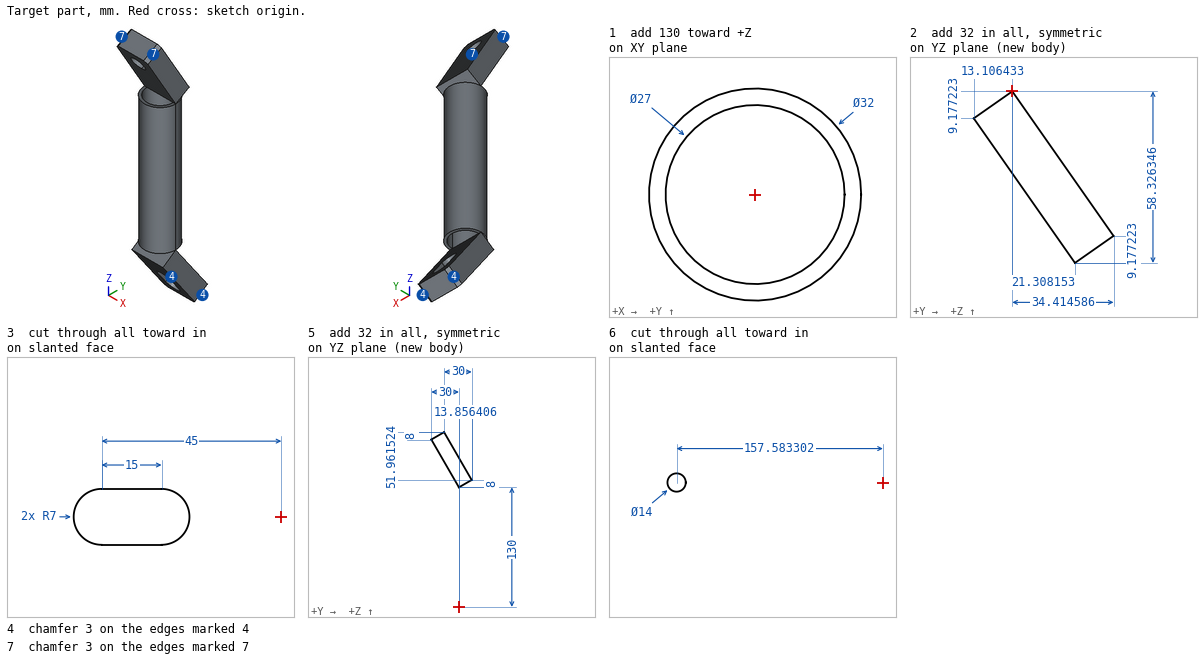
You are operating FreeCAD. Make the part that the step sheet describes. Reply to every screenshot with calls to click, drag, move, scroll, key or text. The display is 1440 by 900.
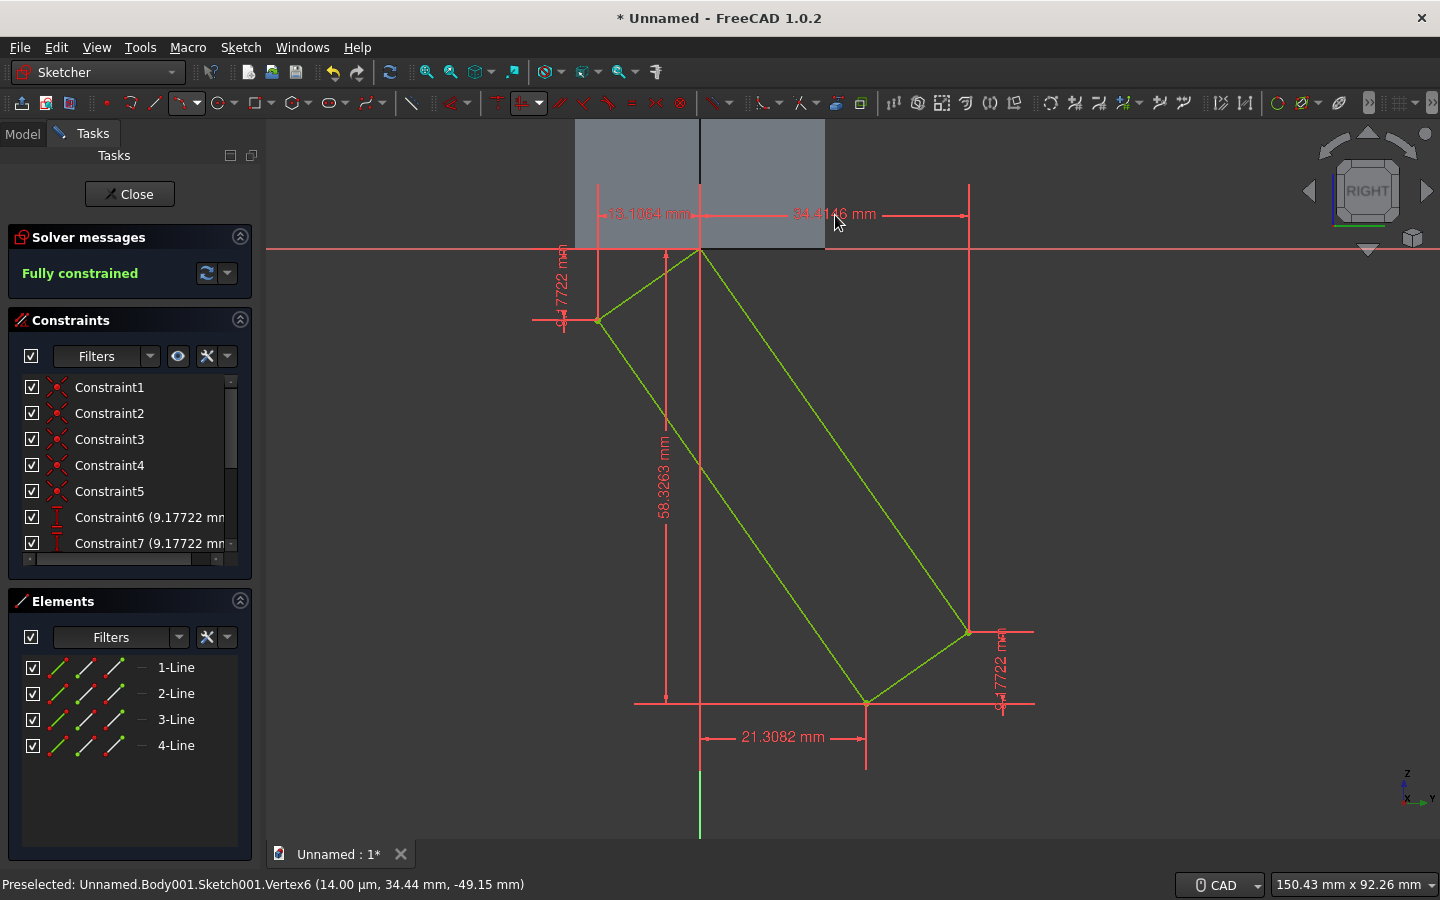
click(130, 194)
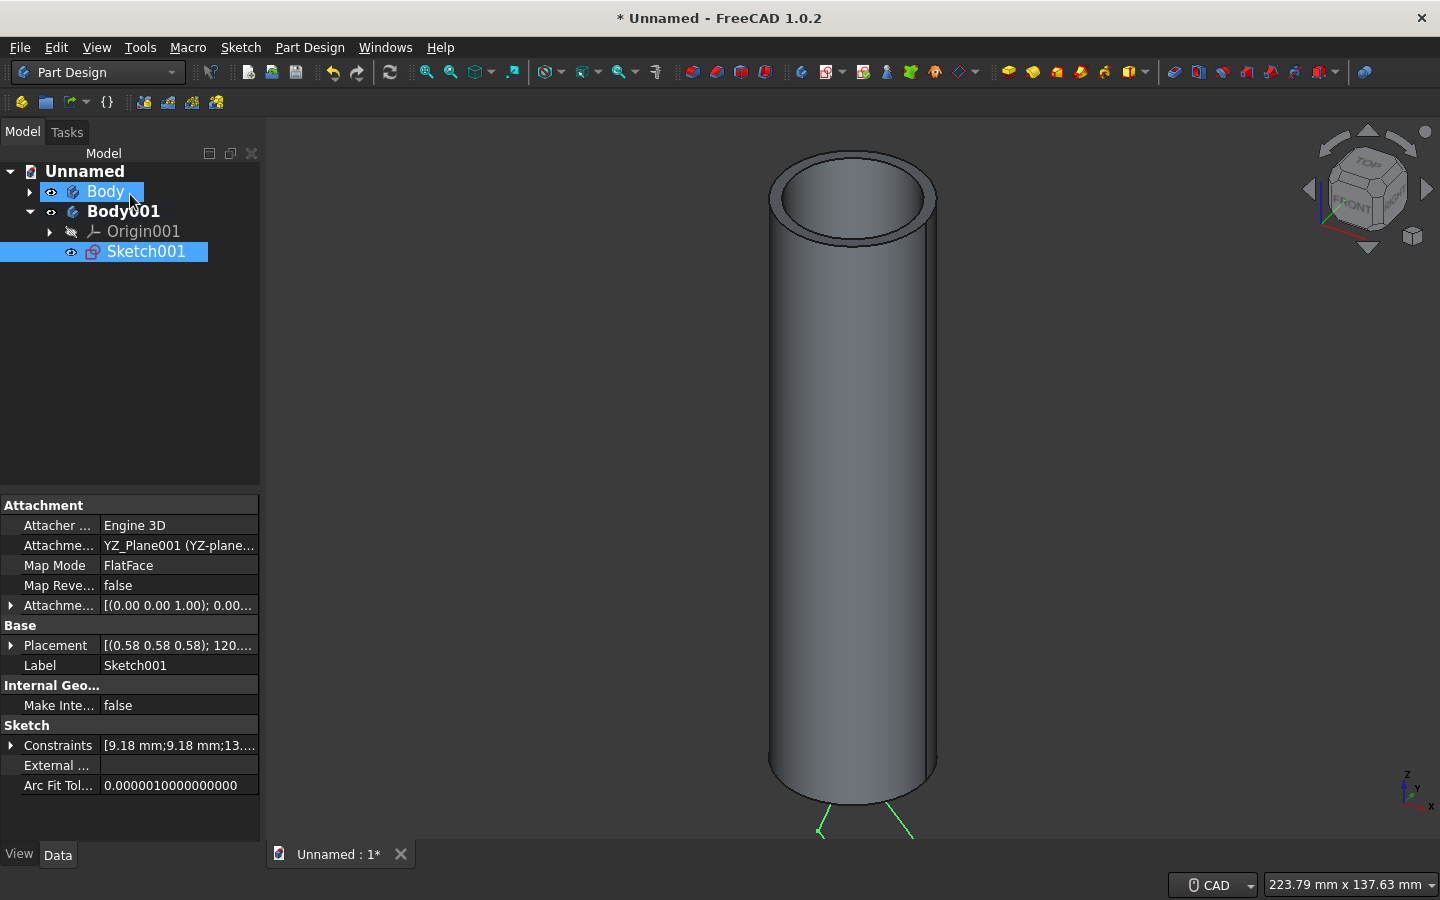
click(1010, 72)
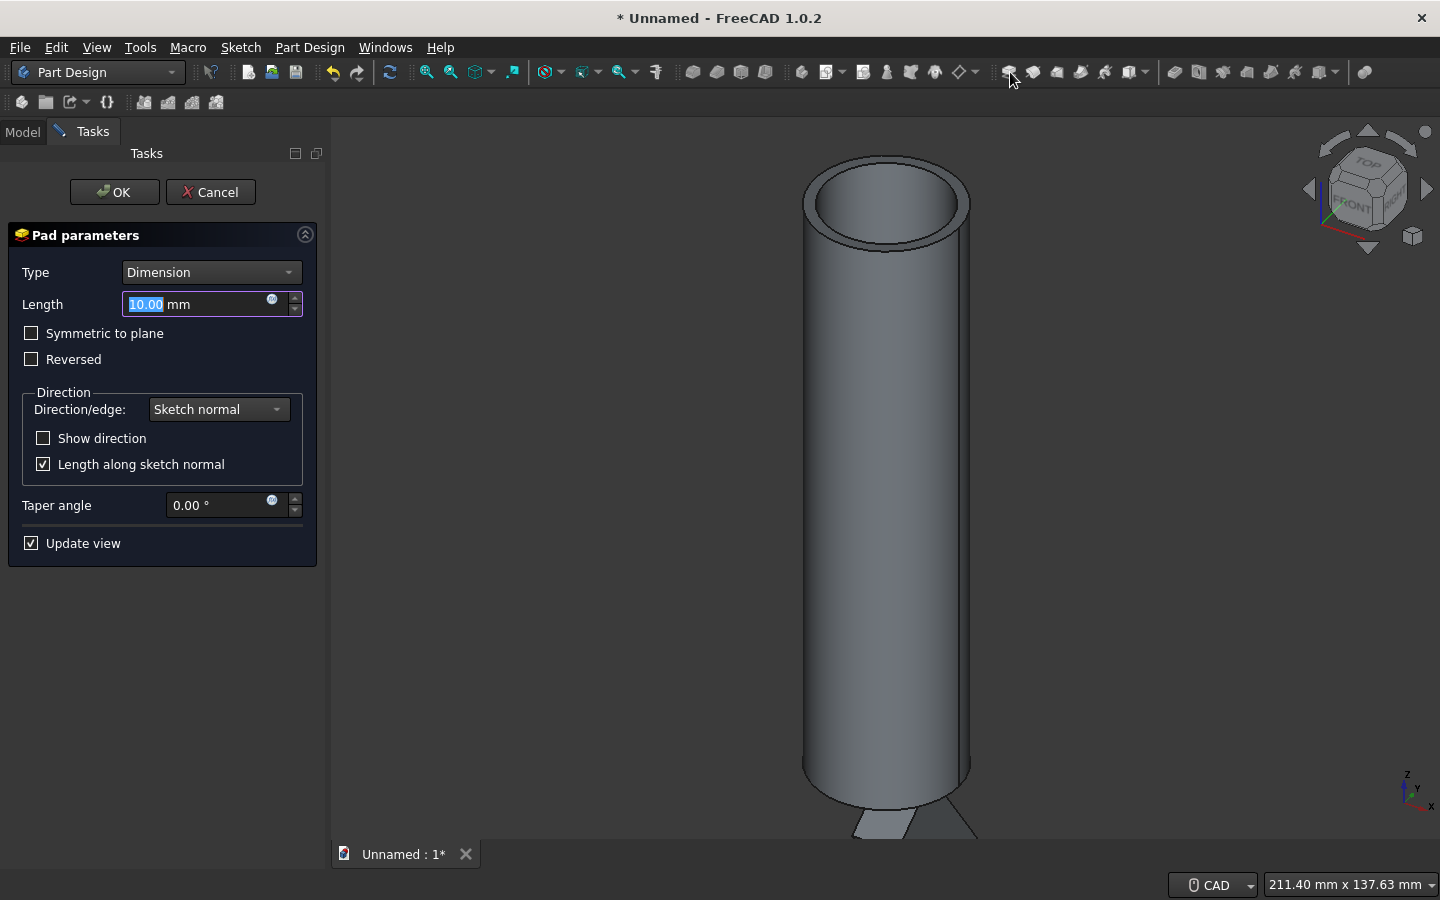
text(32)
key(Tab)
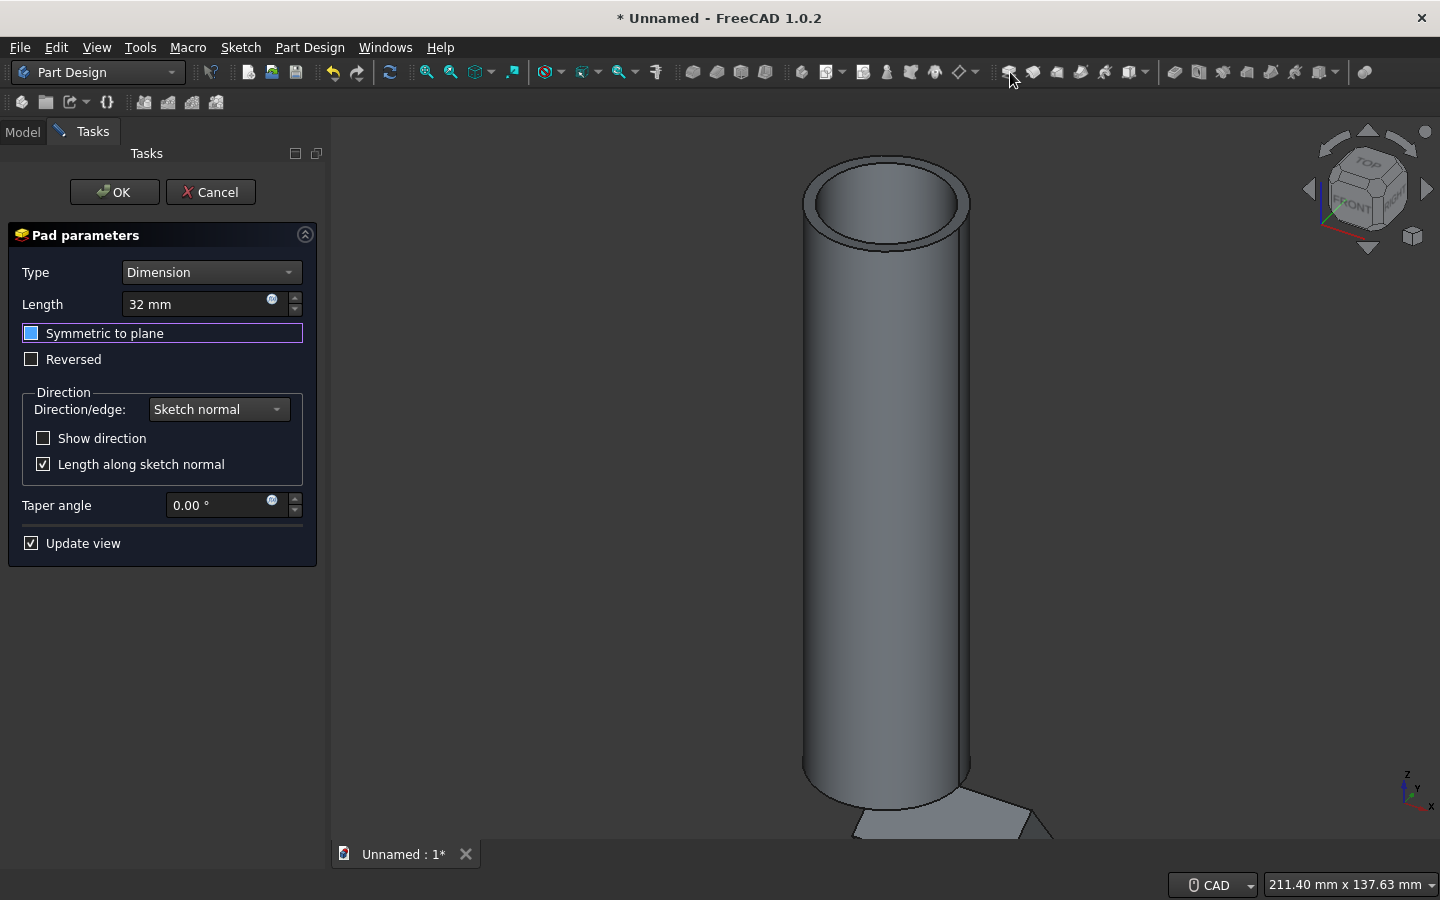
click(30, 333)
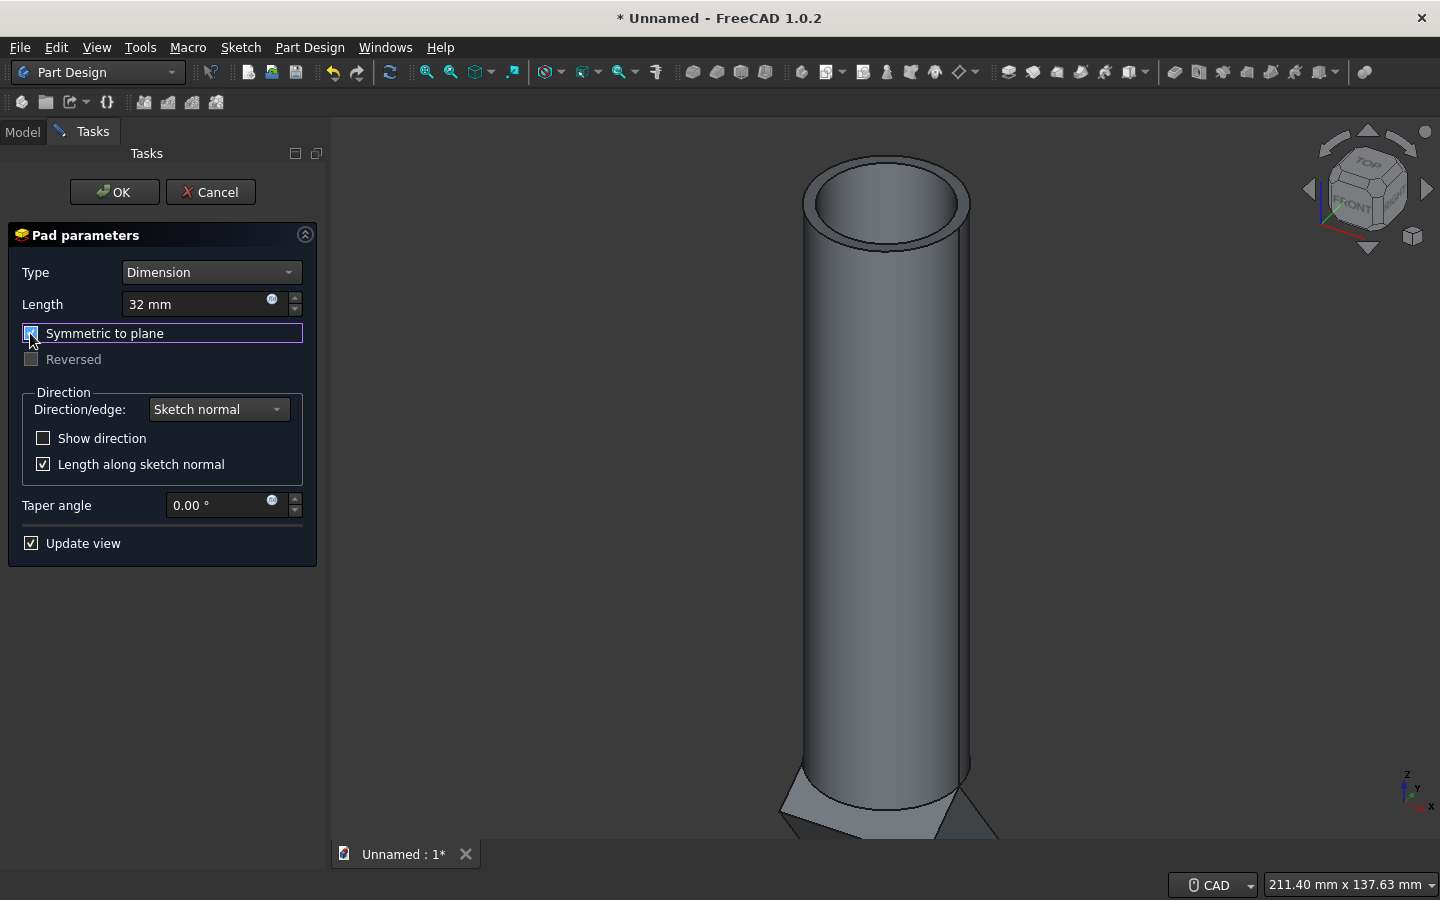
click(115, 192)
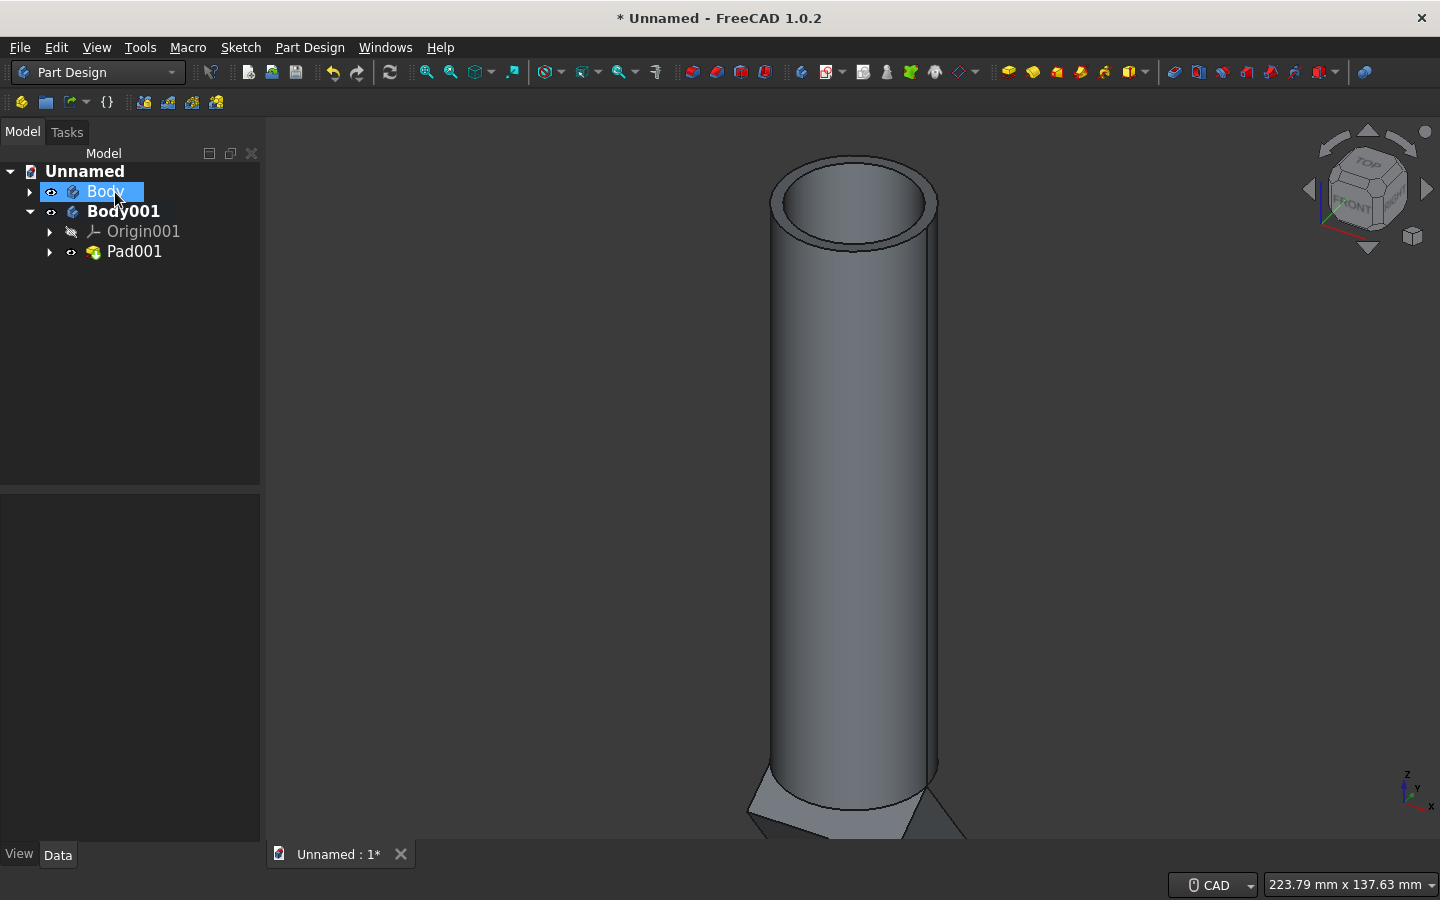
click(428, 72)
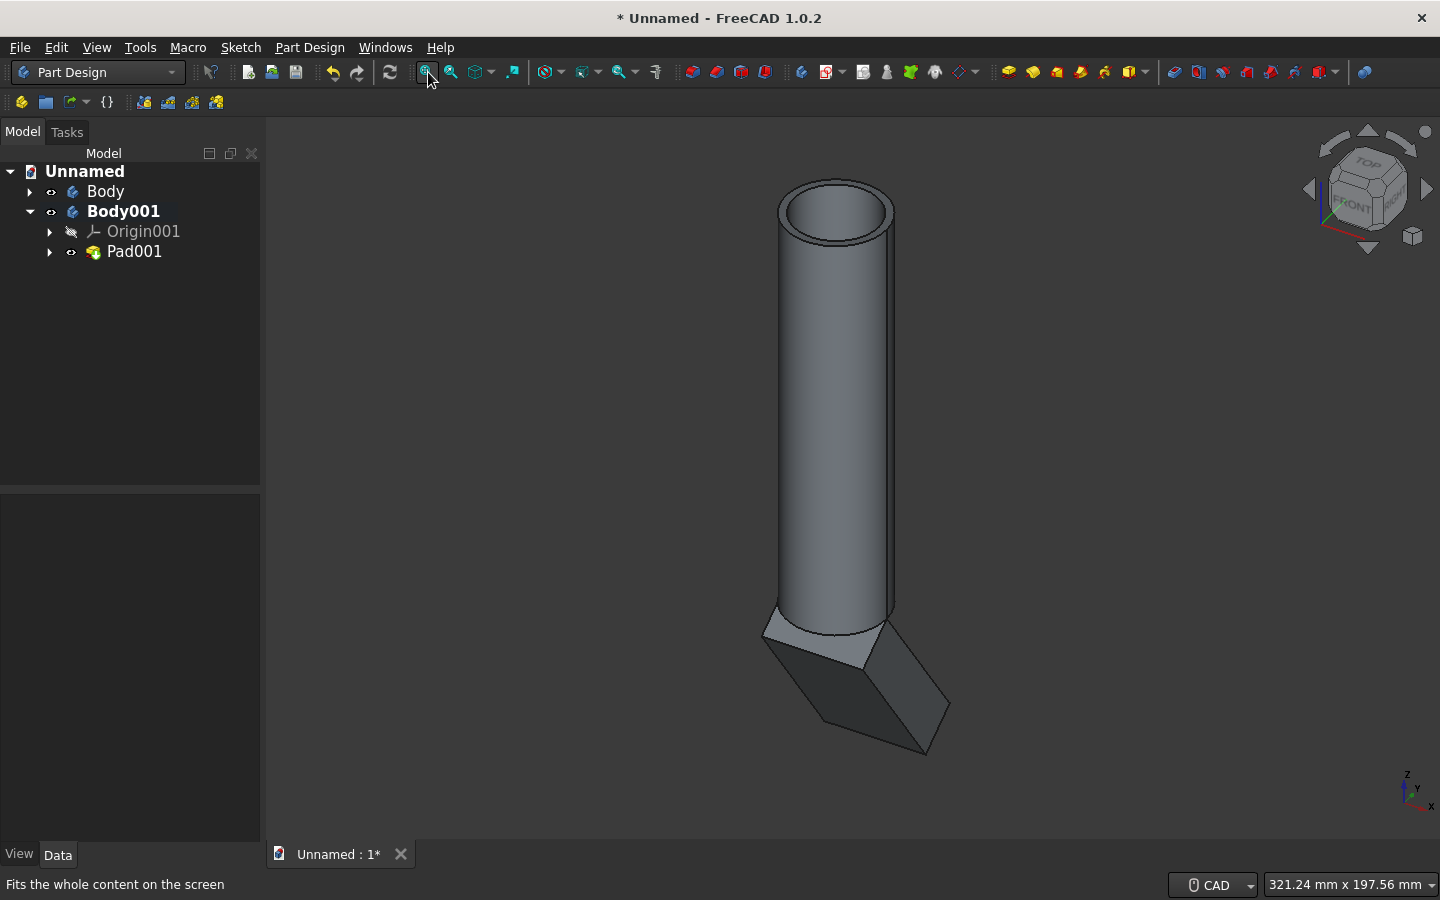
key(4)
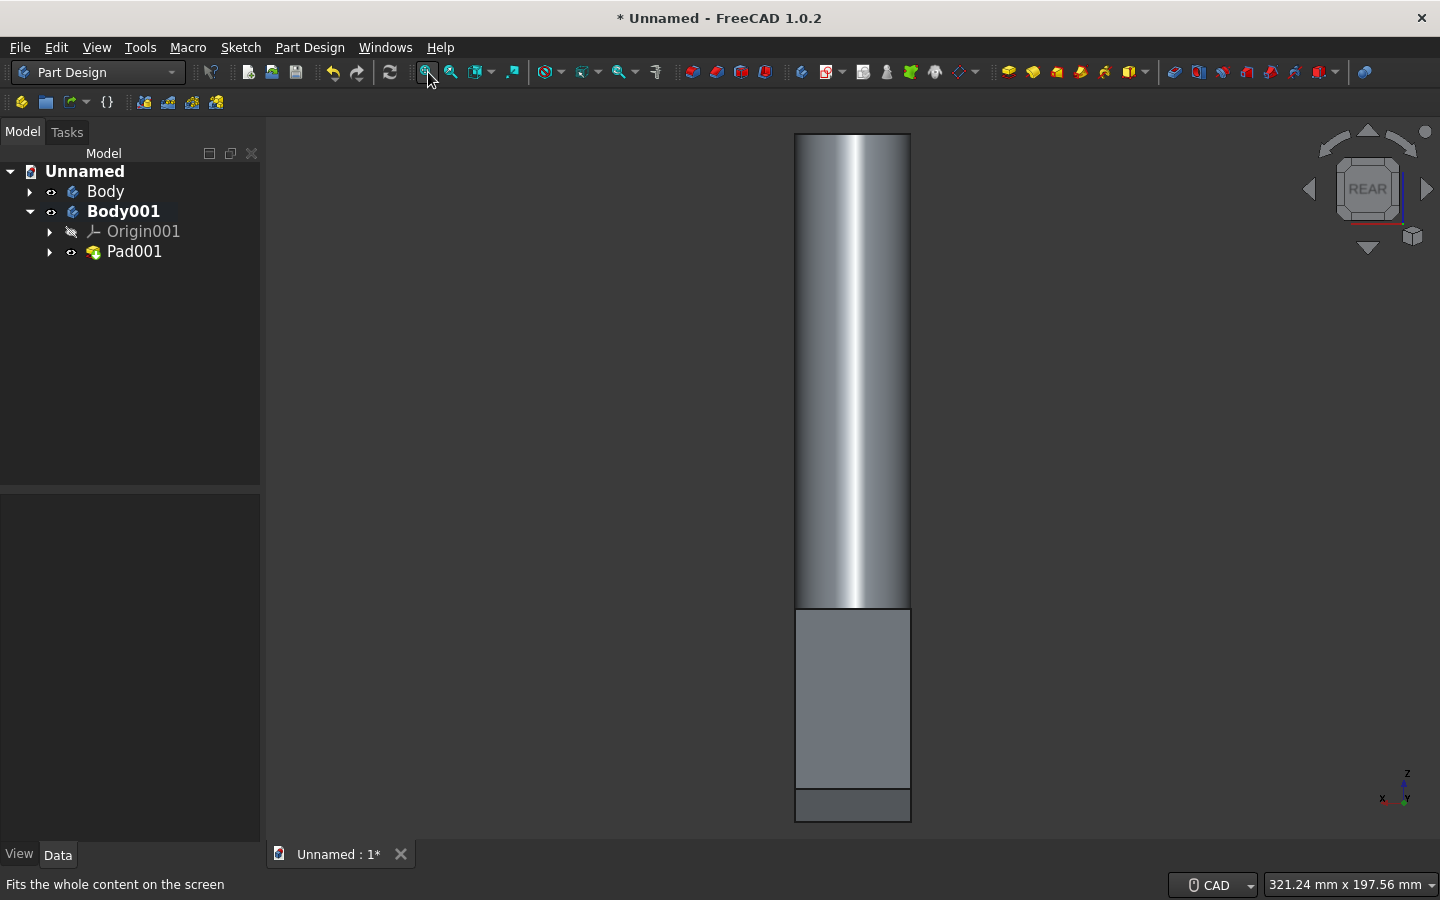
key(v)
key(f)